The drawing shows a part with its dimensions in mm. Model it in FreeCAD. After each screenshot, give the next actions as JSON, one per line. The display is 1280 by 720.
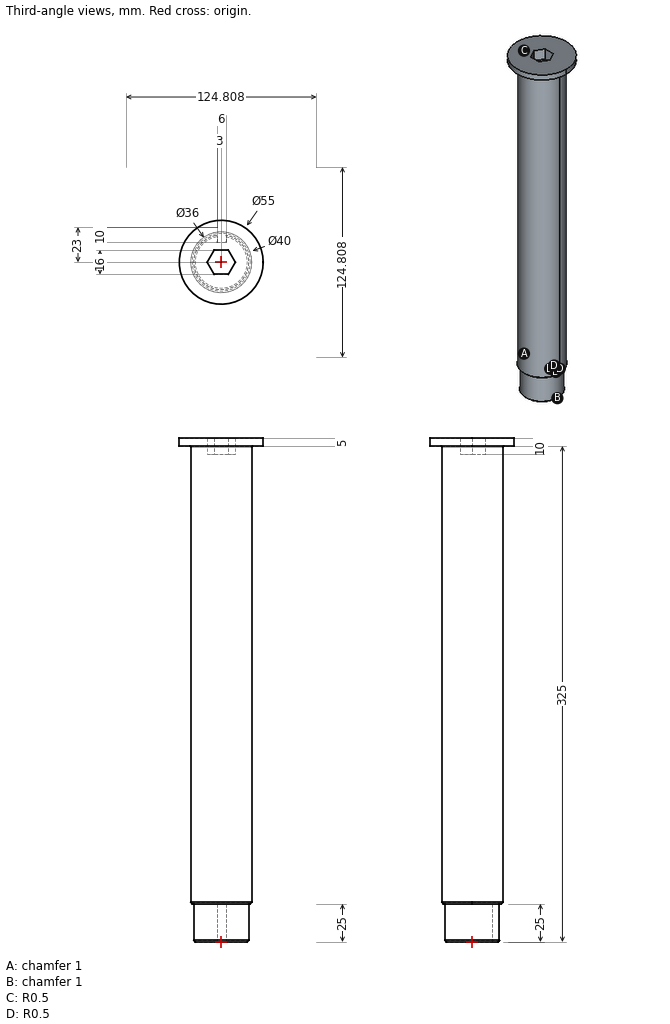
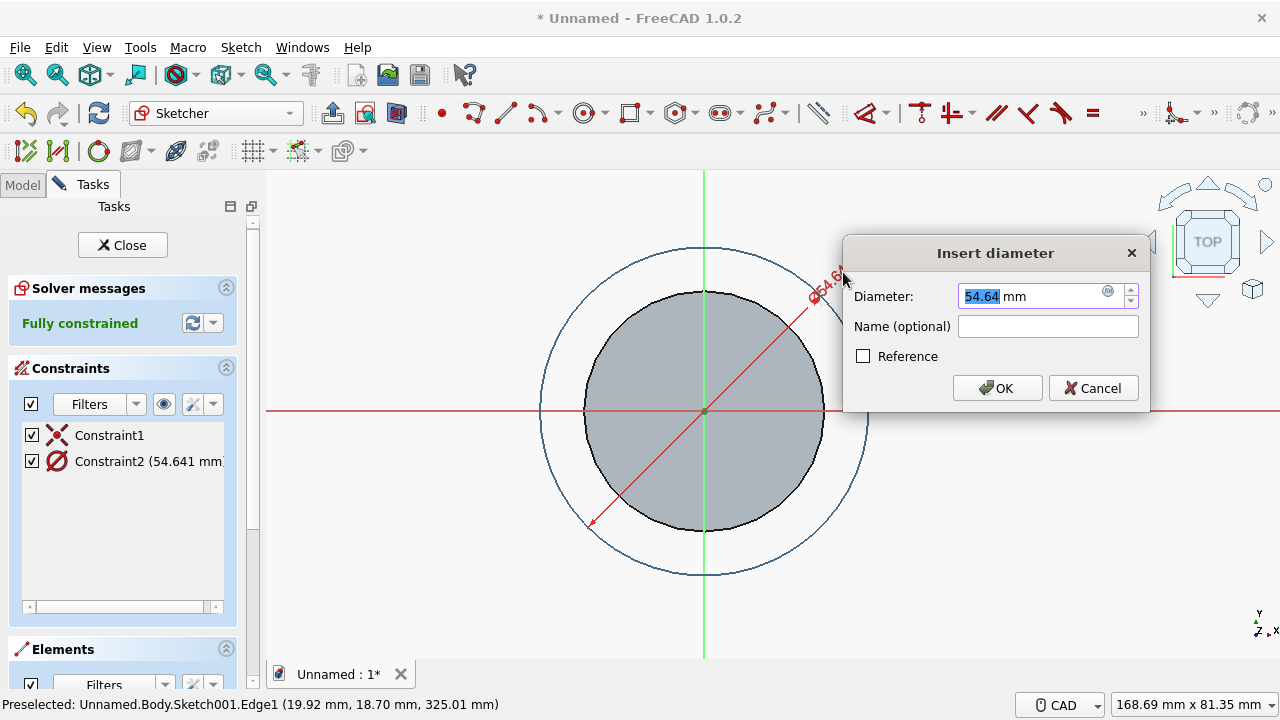
{"action": "type", "text": "55"}
{"action": "key", "text": "Return"}
{"action": "key", "text": "Escape"}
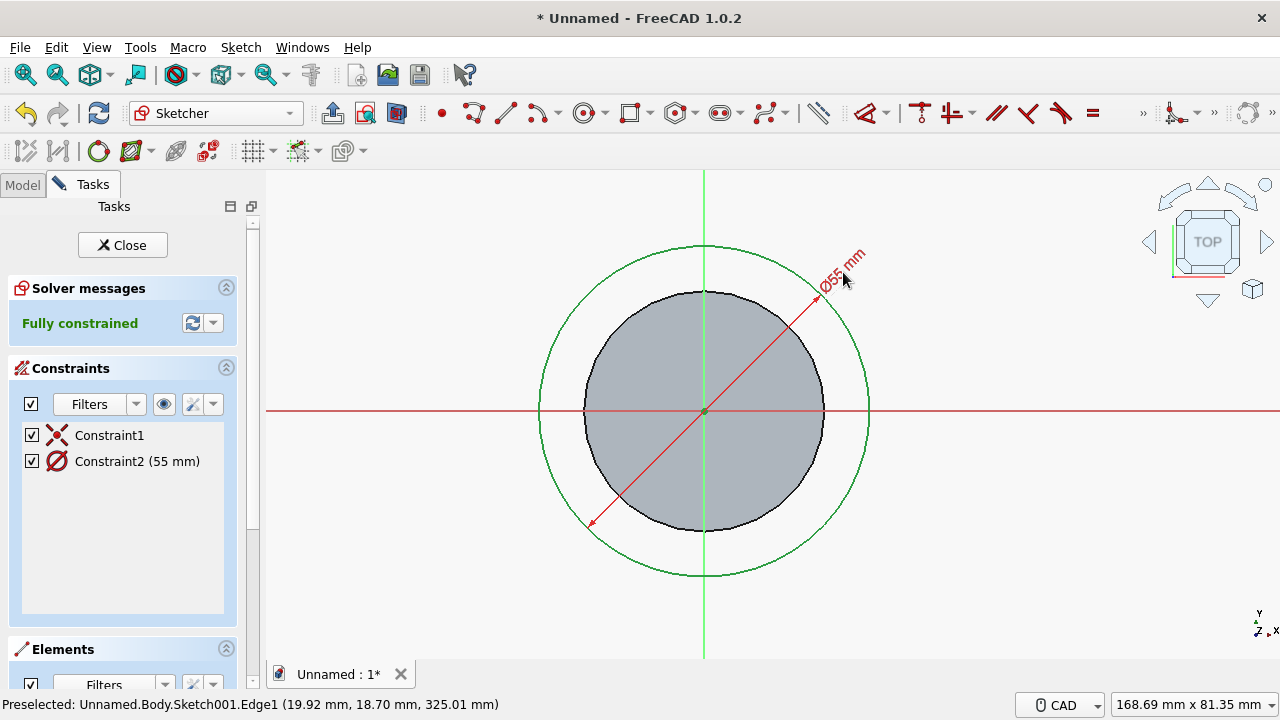
{"action": "left_click", "coordinate": [123, 245]}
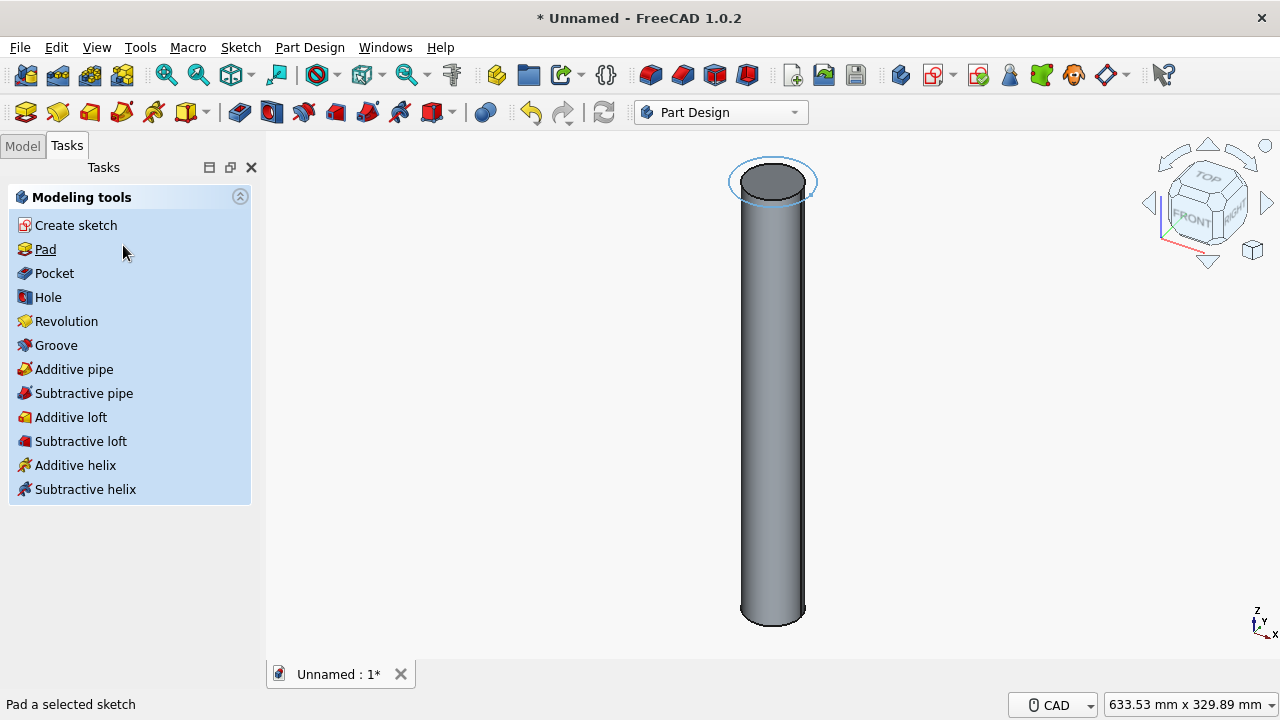
{"action": "left_click", "coordinate": [26, 112]}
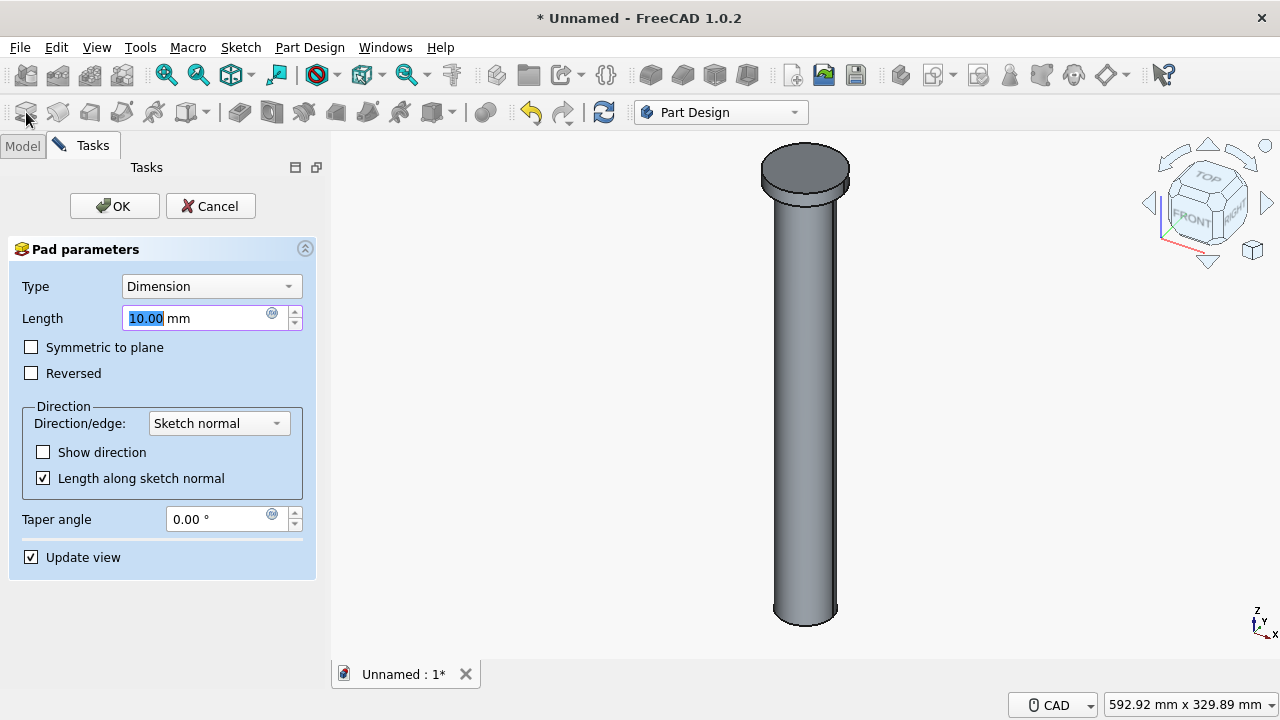
{"action": "type", "text": "5"}
{"action": "key", "text": "Tab"}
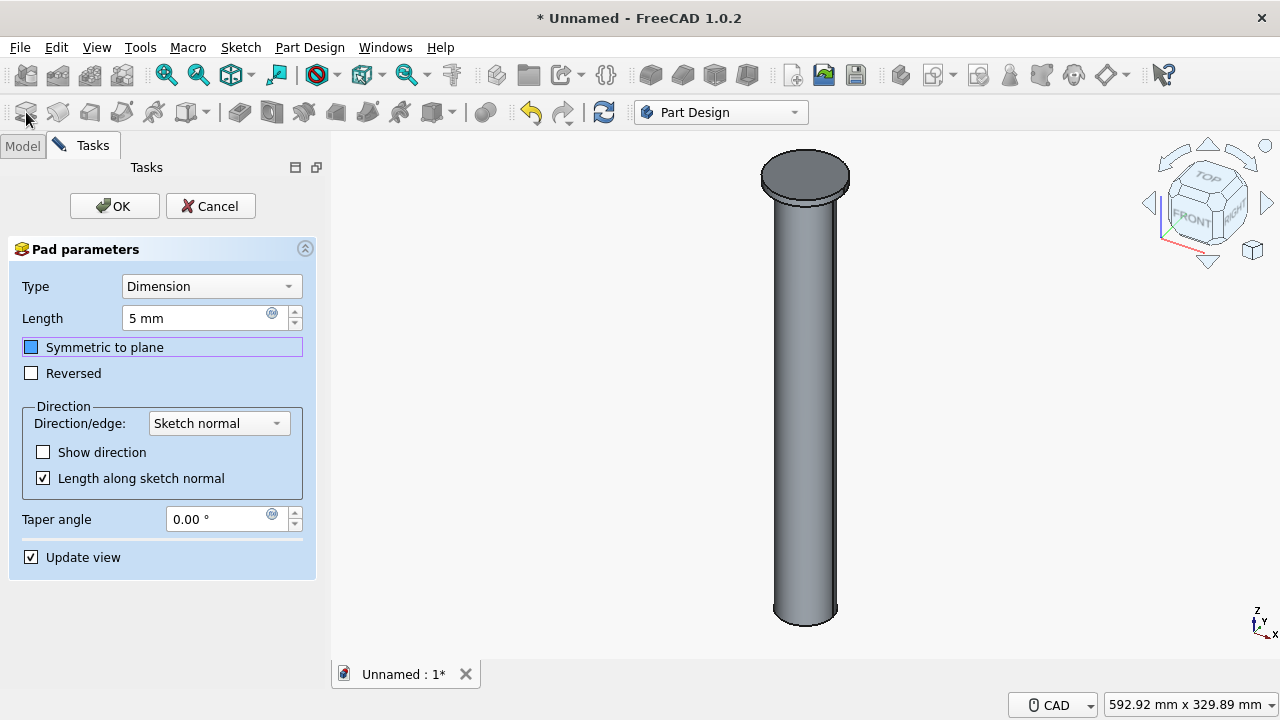
{"action": "left_click", "coordinate": [115, 206]}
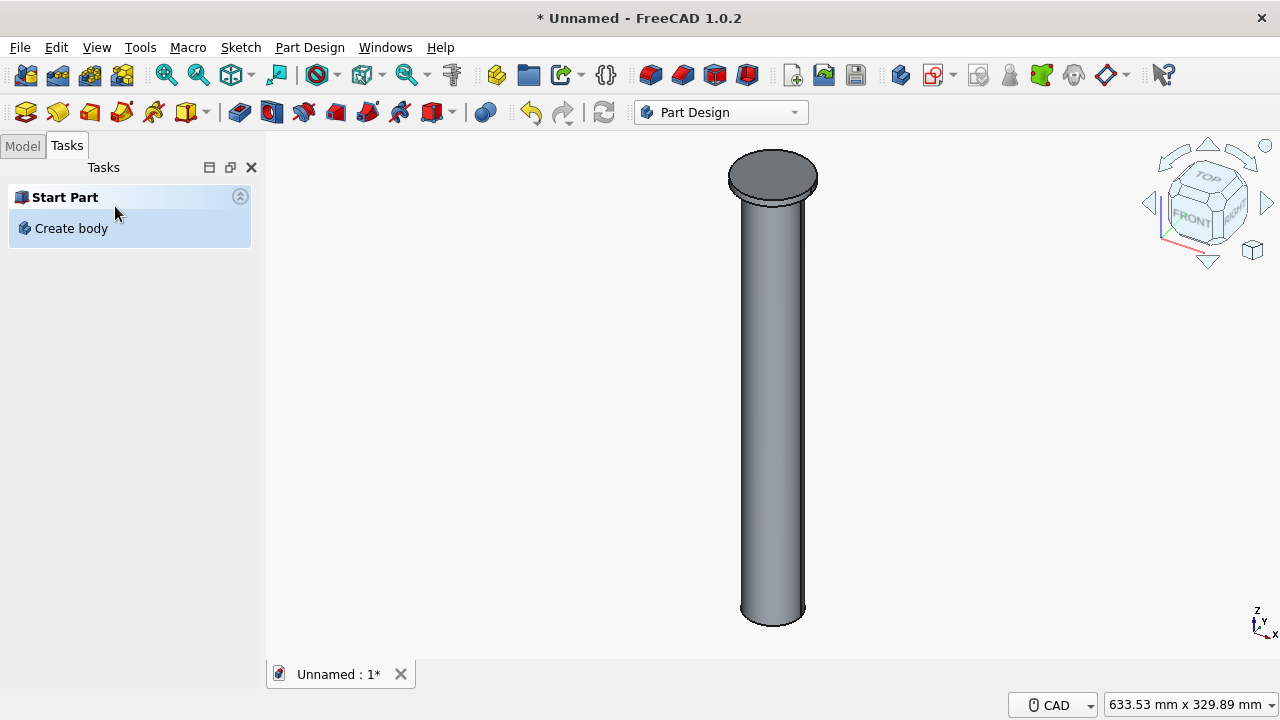
{"action": "left_click", "coordinate": [773, 174]}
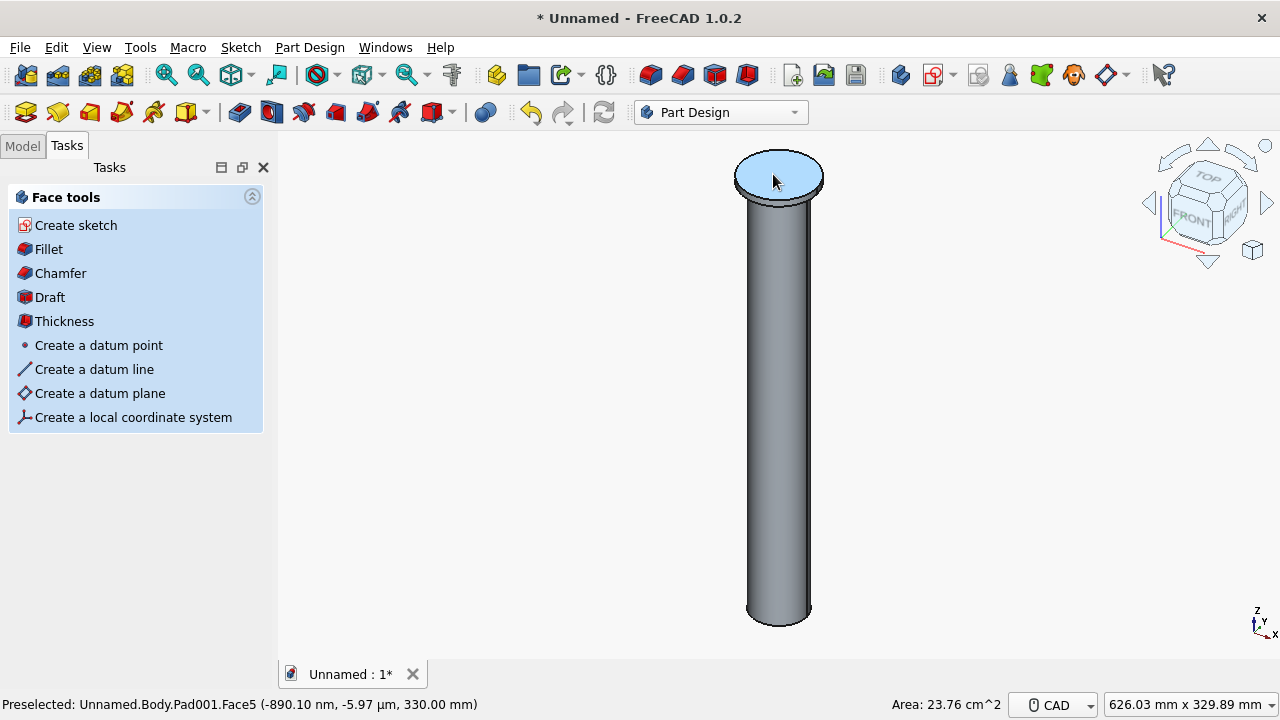
{"action": "left_click", "coordinate": [934, 76]}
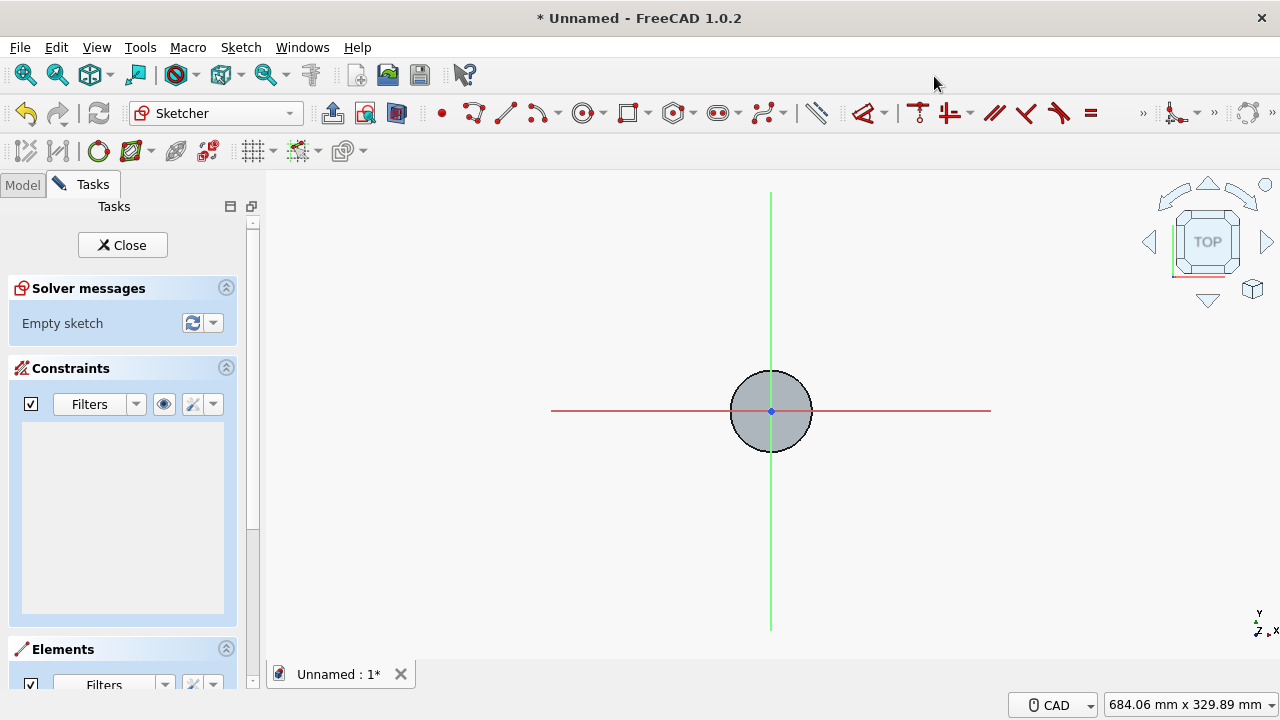
{"action": "scroll", "coordinate": [777, 411], "scroll_direction": "up", "scroll_amount": 13}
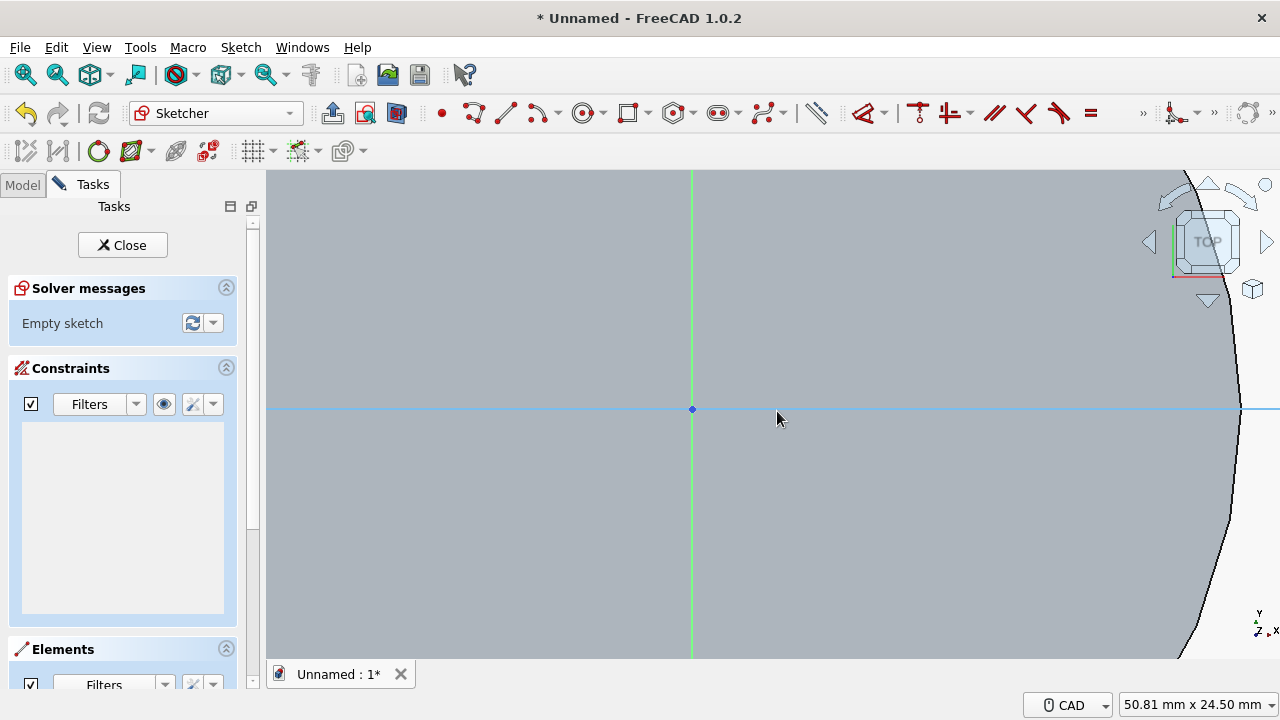
{"action": "left_click", "coordinate": [674, 114]}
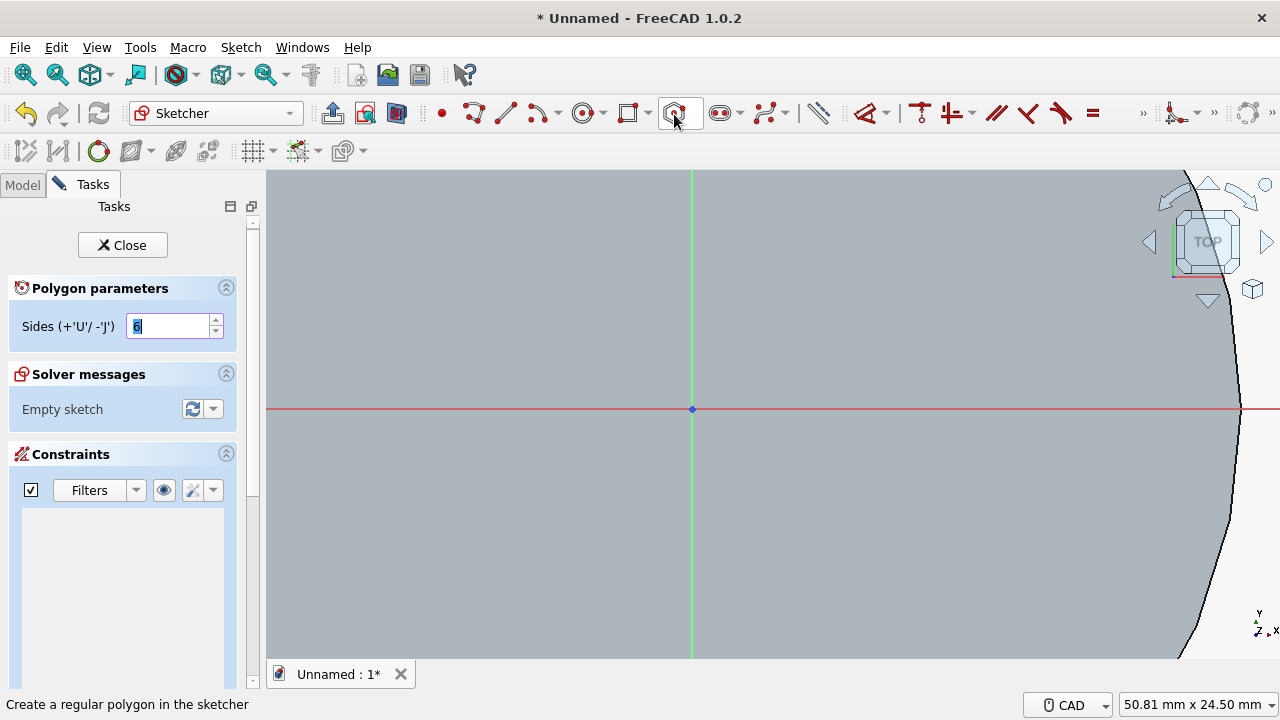
{"action": "left_click", "coordinate": [692, 409]}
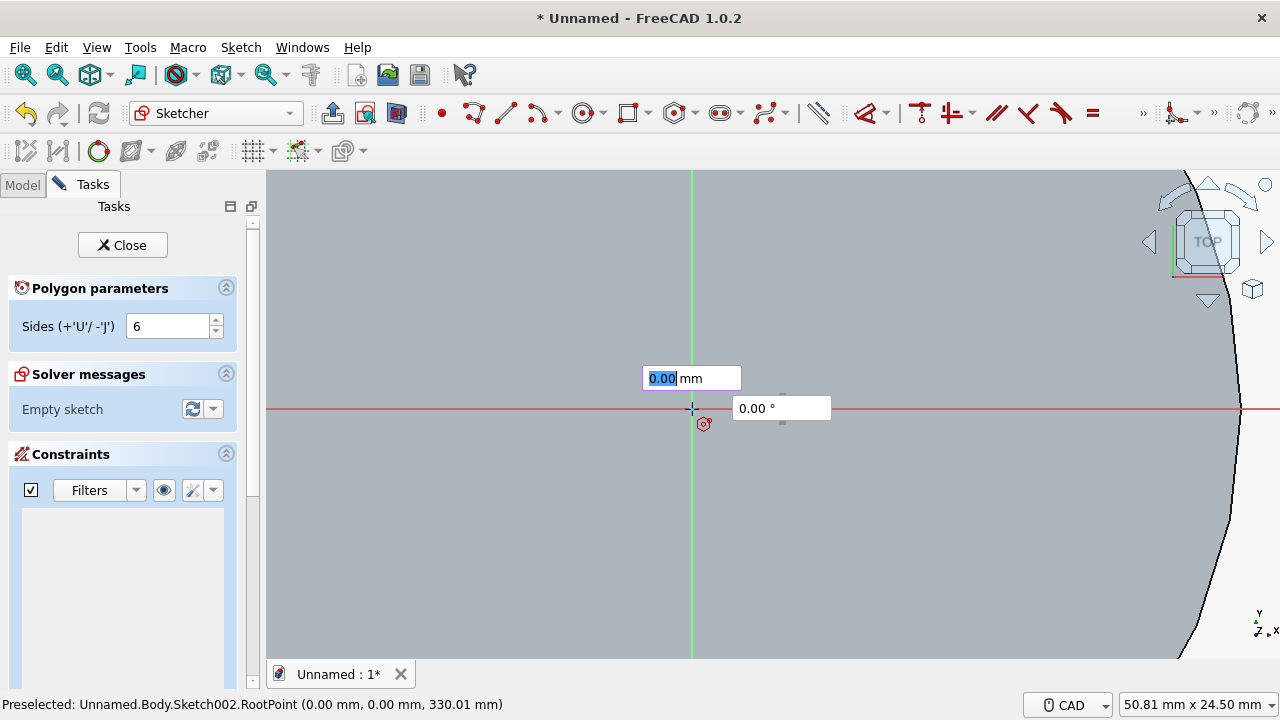
{"action": "left_click", "coordinate": [877, 409]}
{"action": "right_click", "coordinate": [877, 409]}